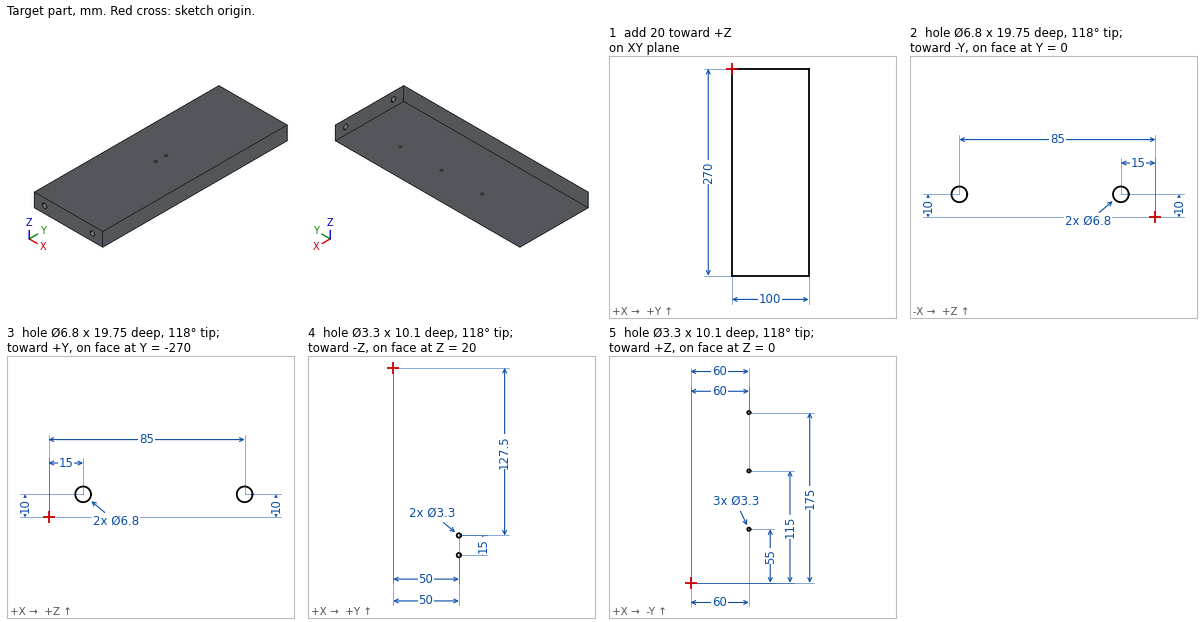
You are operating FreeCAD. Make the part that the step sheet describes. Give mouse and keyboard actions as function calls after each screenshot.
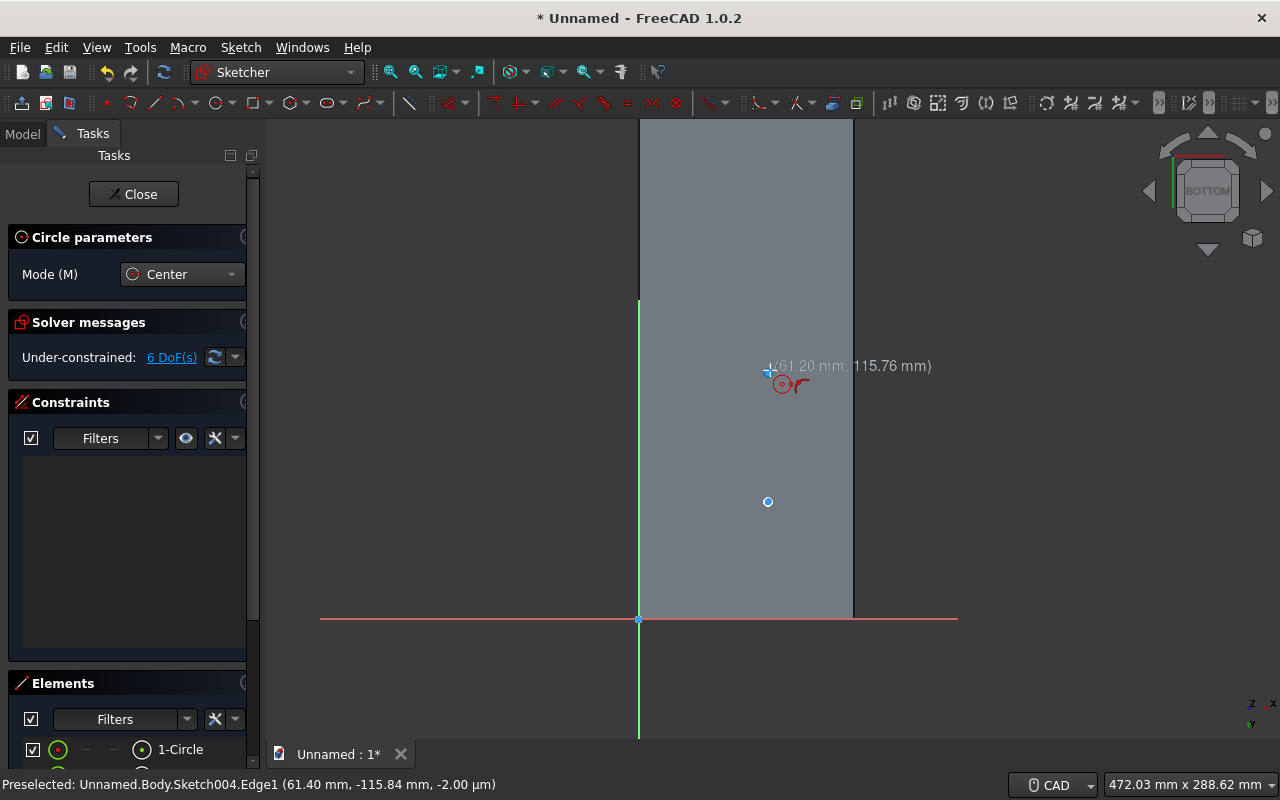
scroll(768, 243, up, 10)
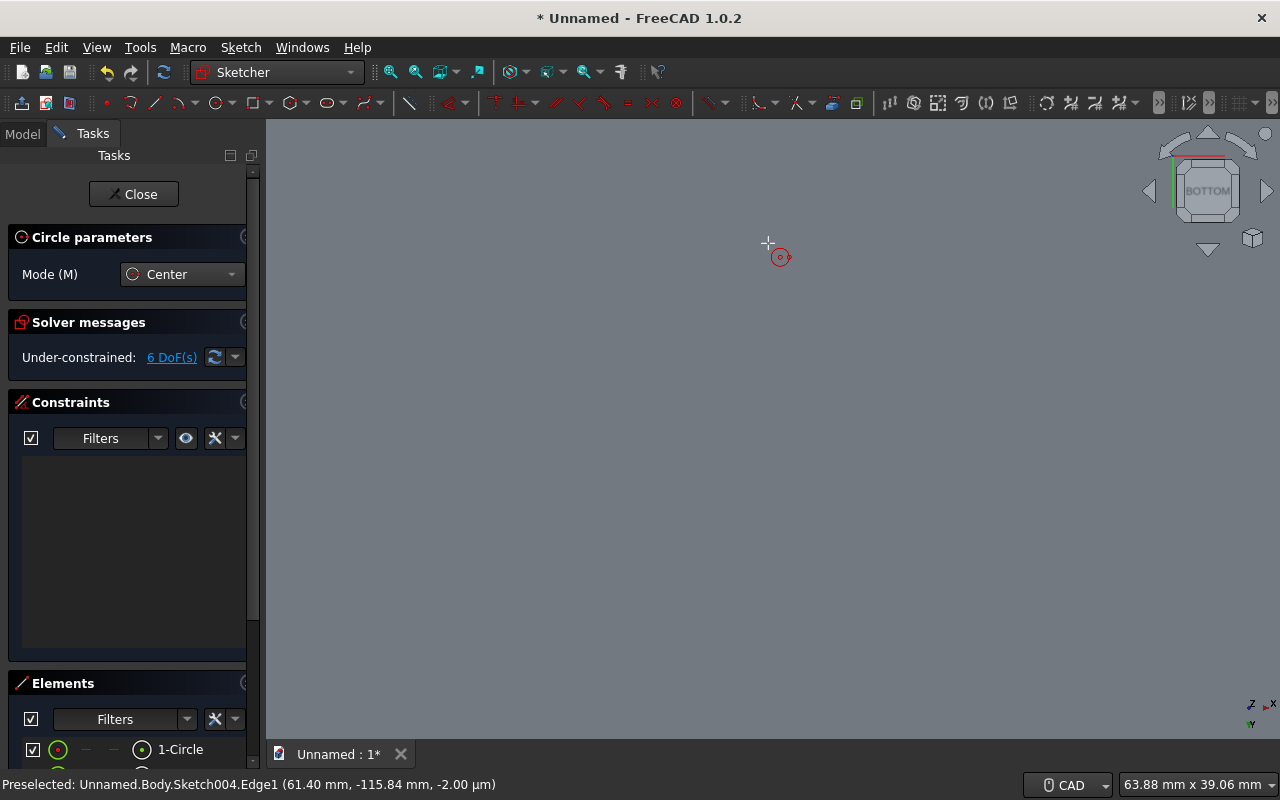
scroll(768, 243, down, 10)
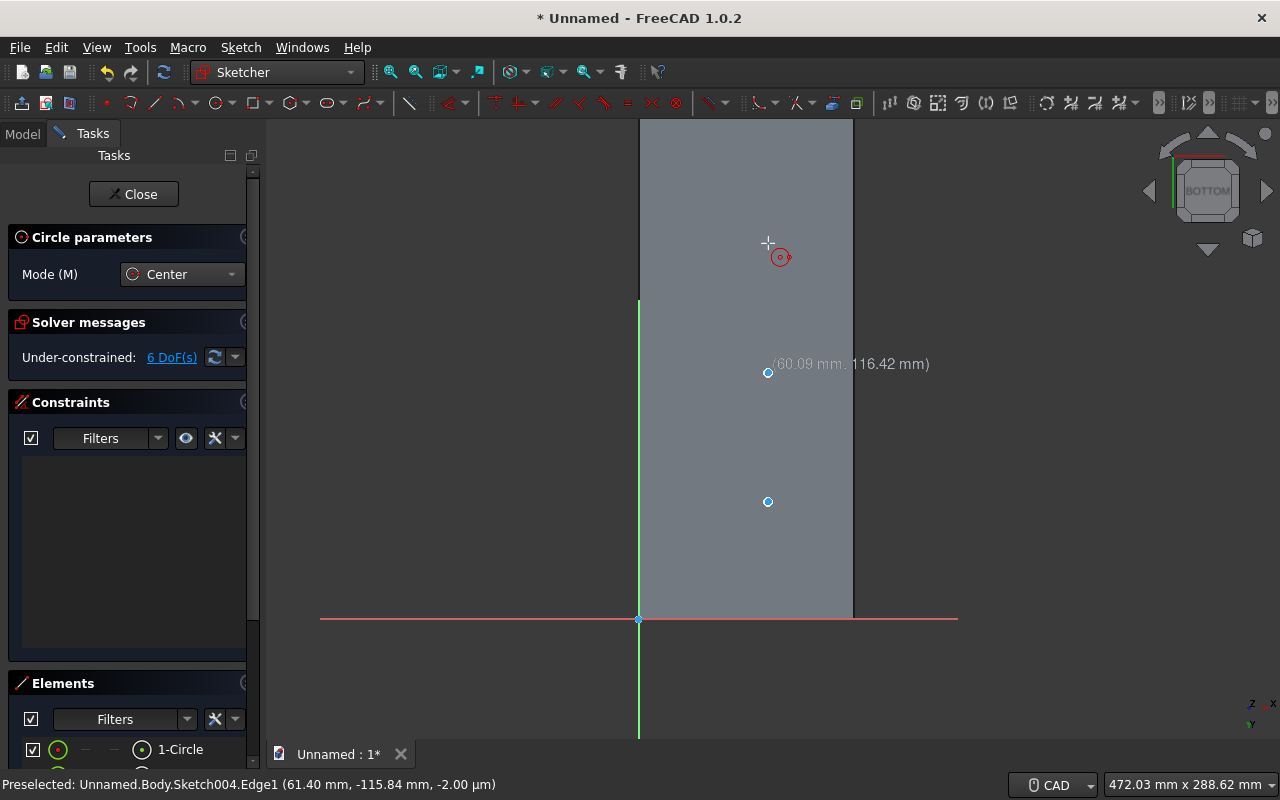
click(768, 243)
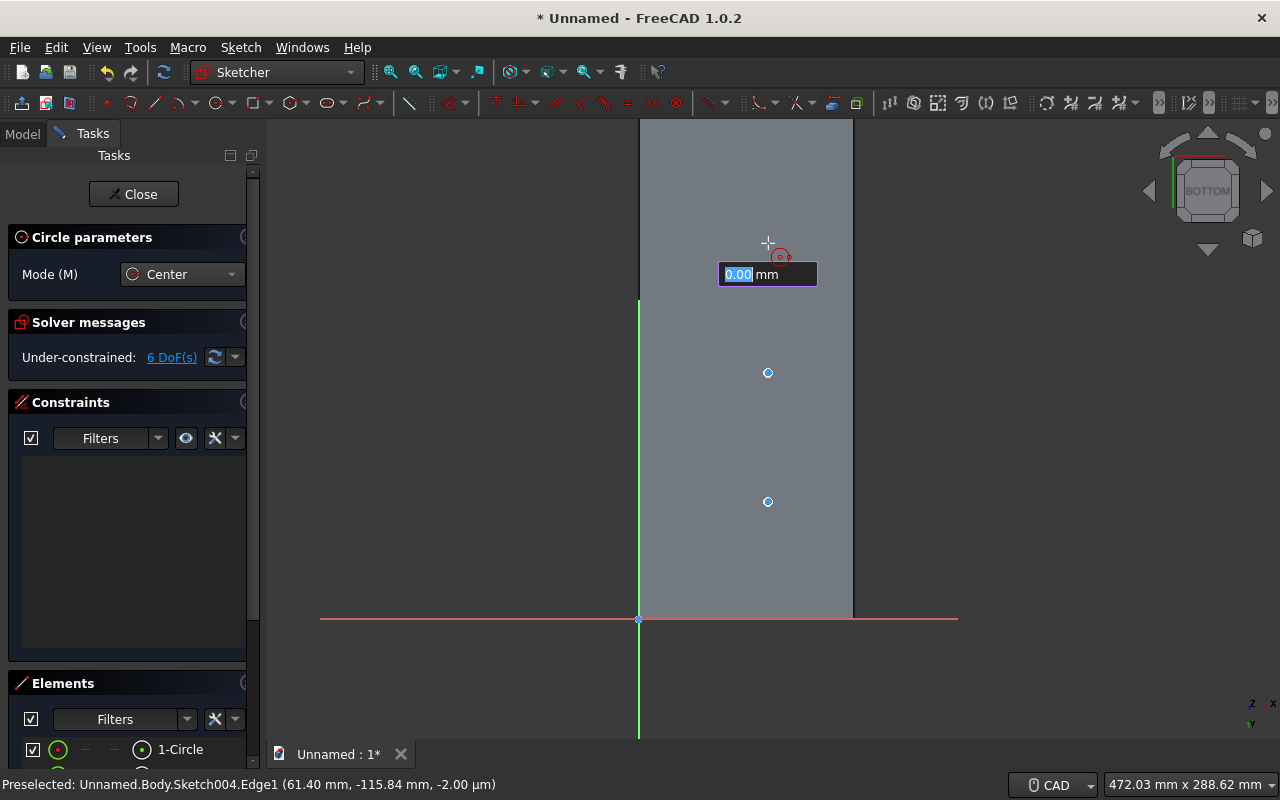
scroll(770, 241, up, 8)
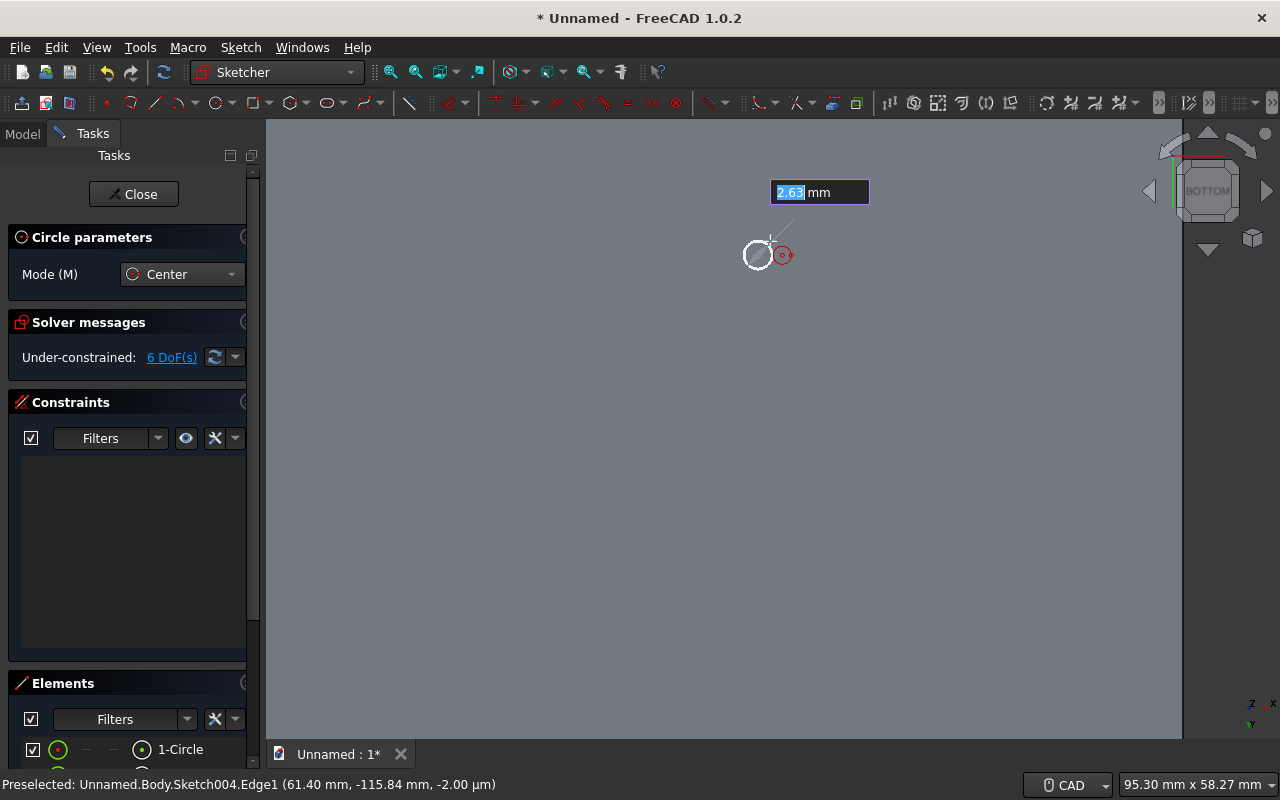
click(770, 239)
key(Escape)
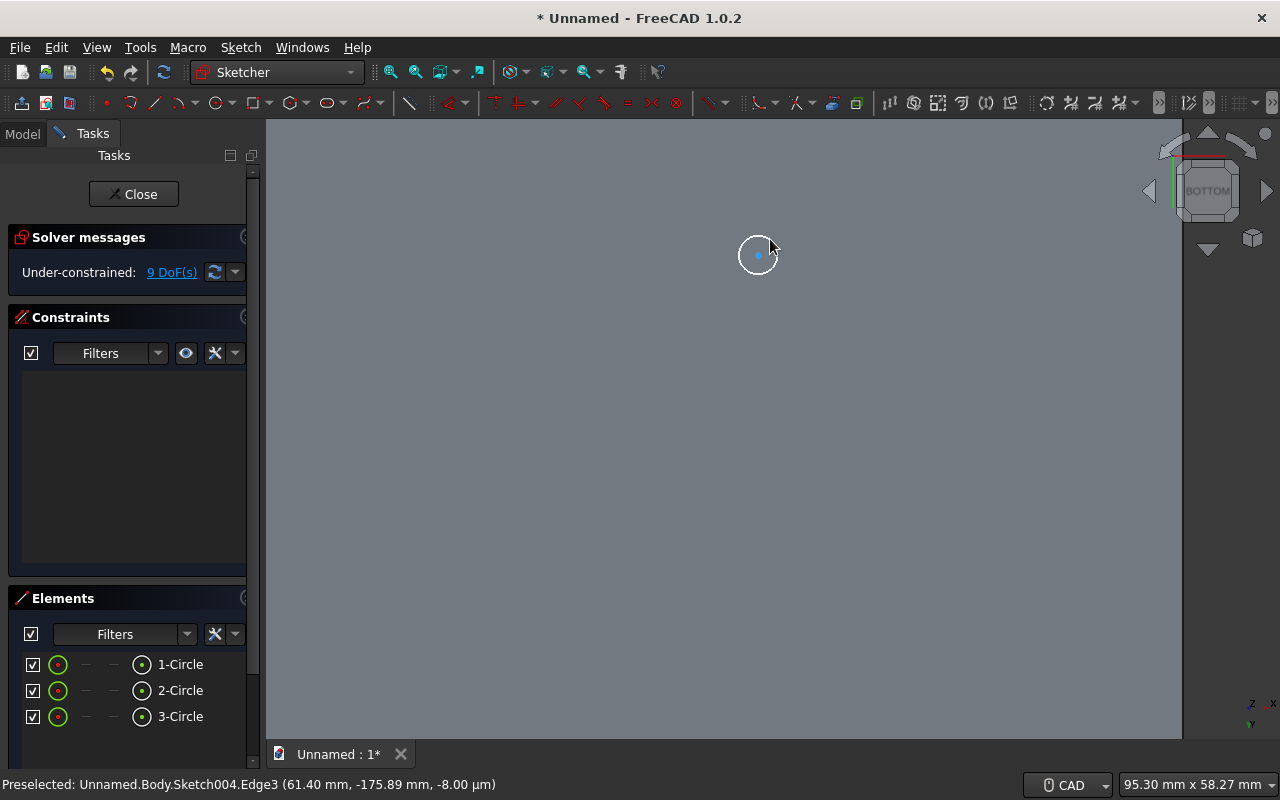
scroll(770, 241, down, 8)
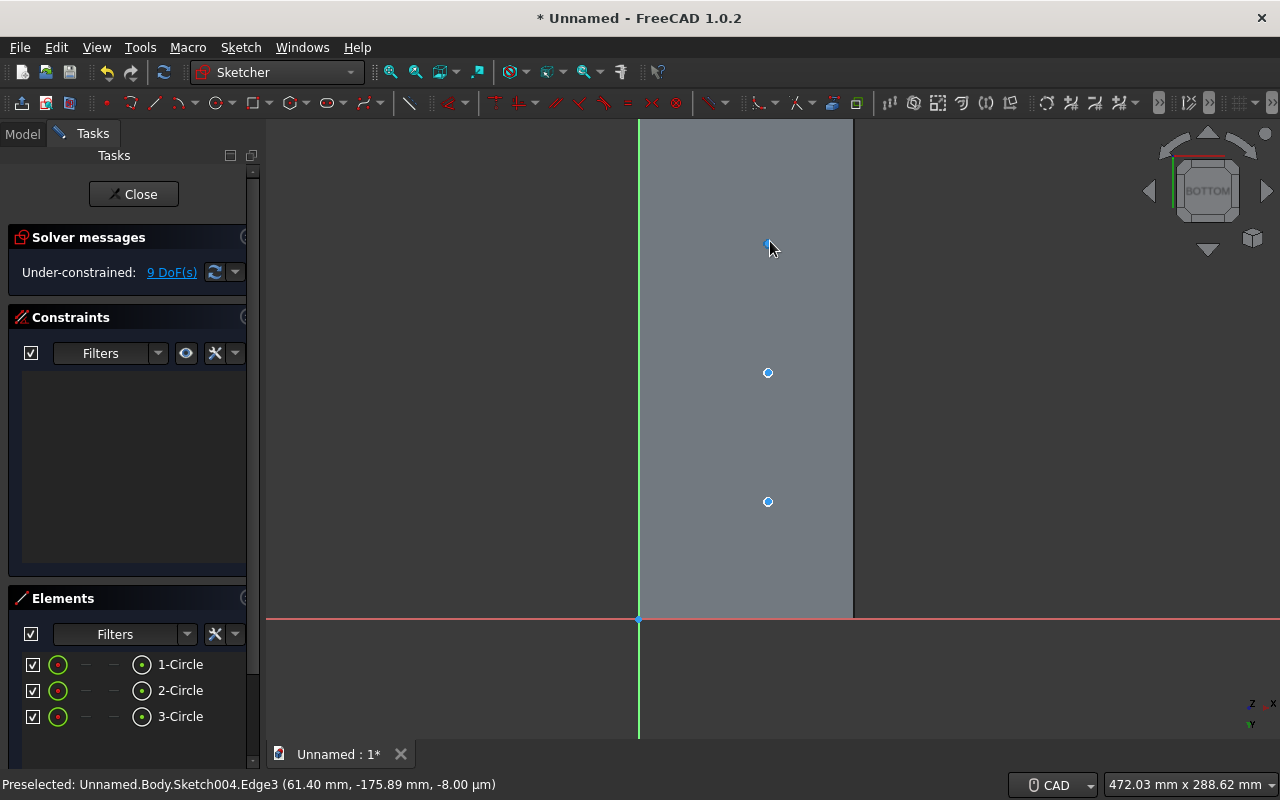
scroll(771, 499, up, 7)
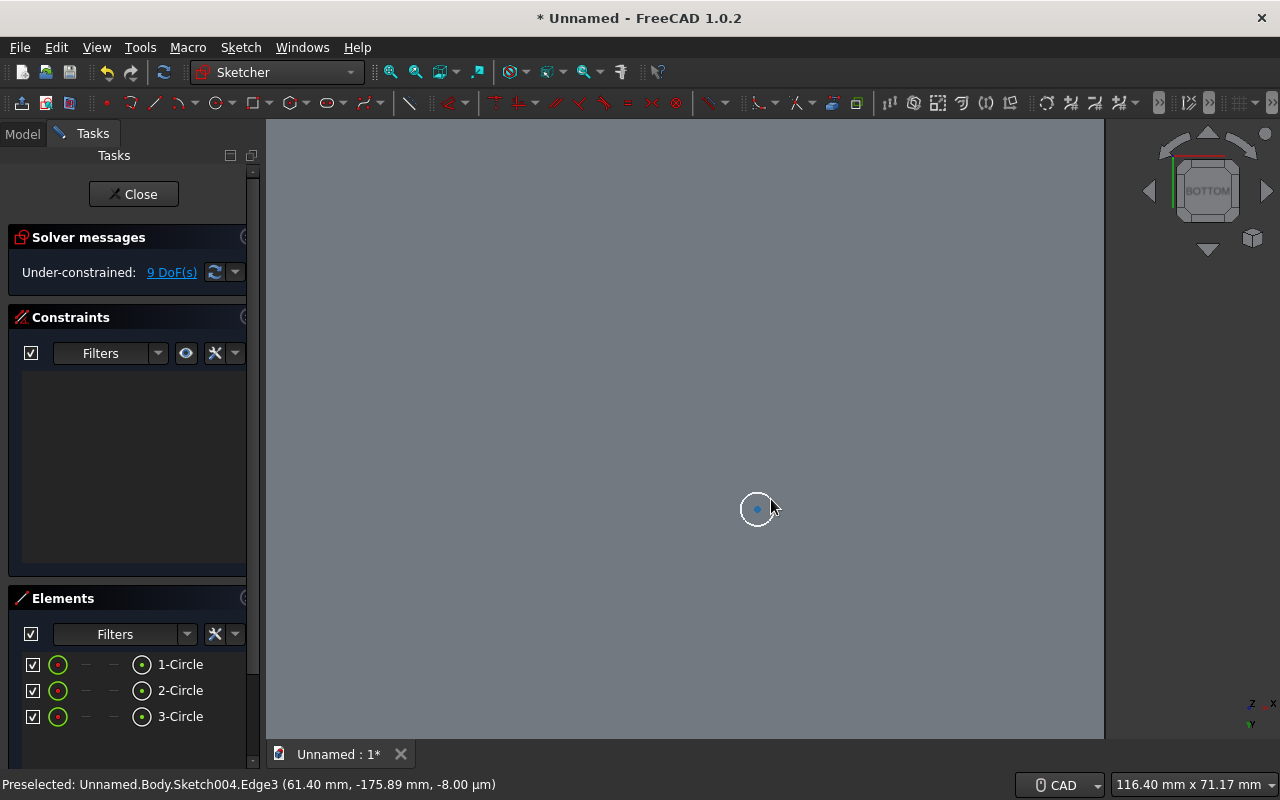
click(769, 498)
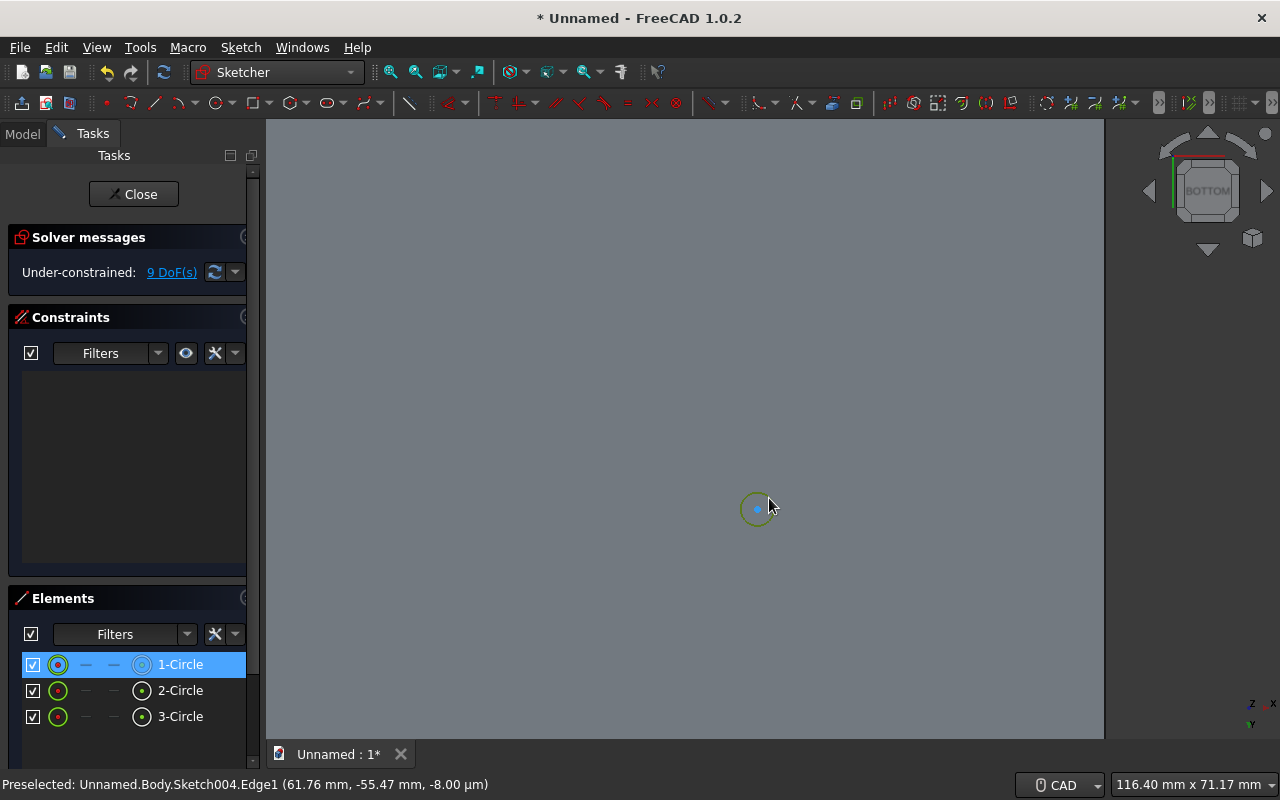
scroll(771, 499, down, 7)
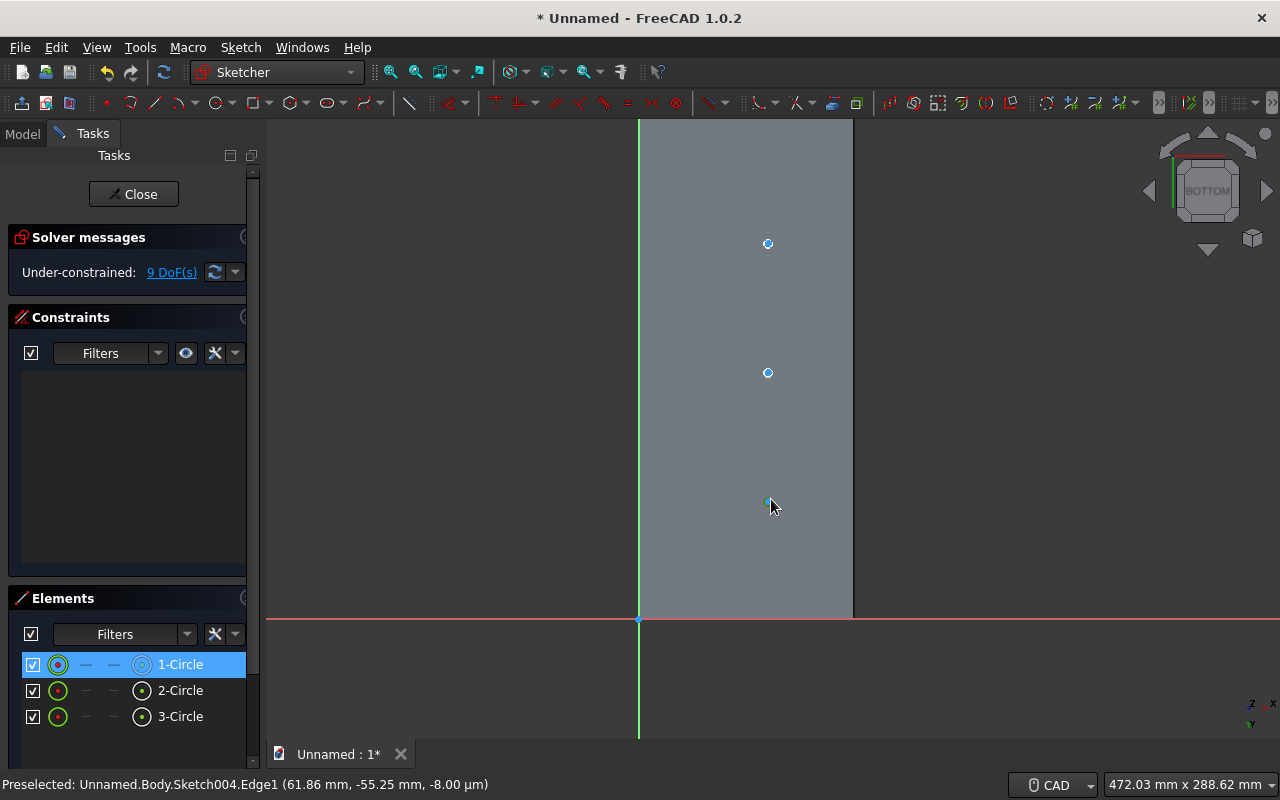
scroll(771, 370, up, 7)